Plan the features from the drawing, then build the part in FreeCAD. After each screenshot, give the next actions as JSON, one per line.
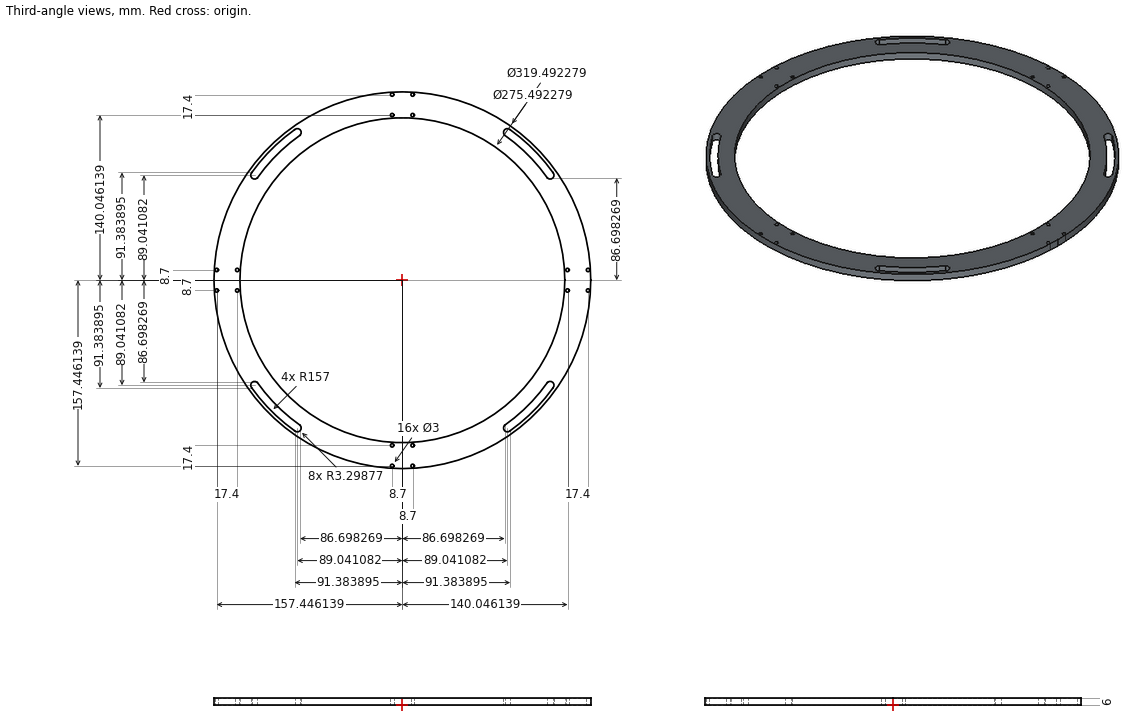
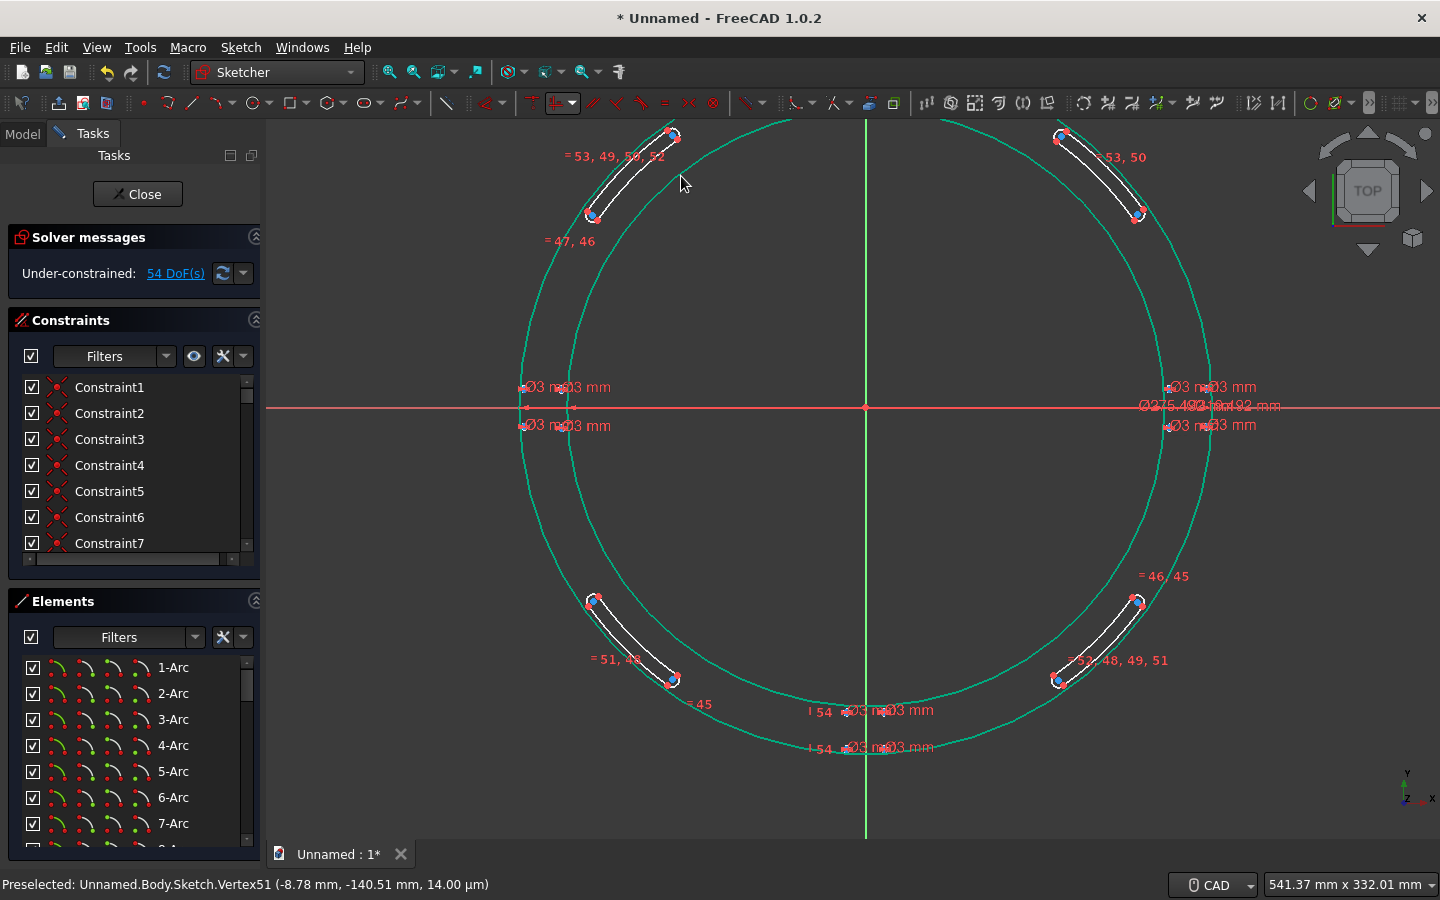
{"action": "left_click", "coordinate": [524, 427]}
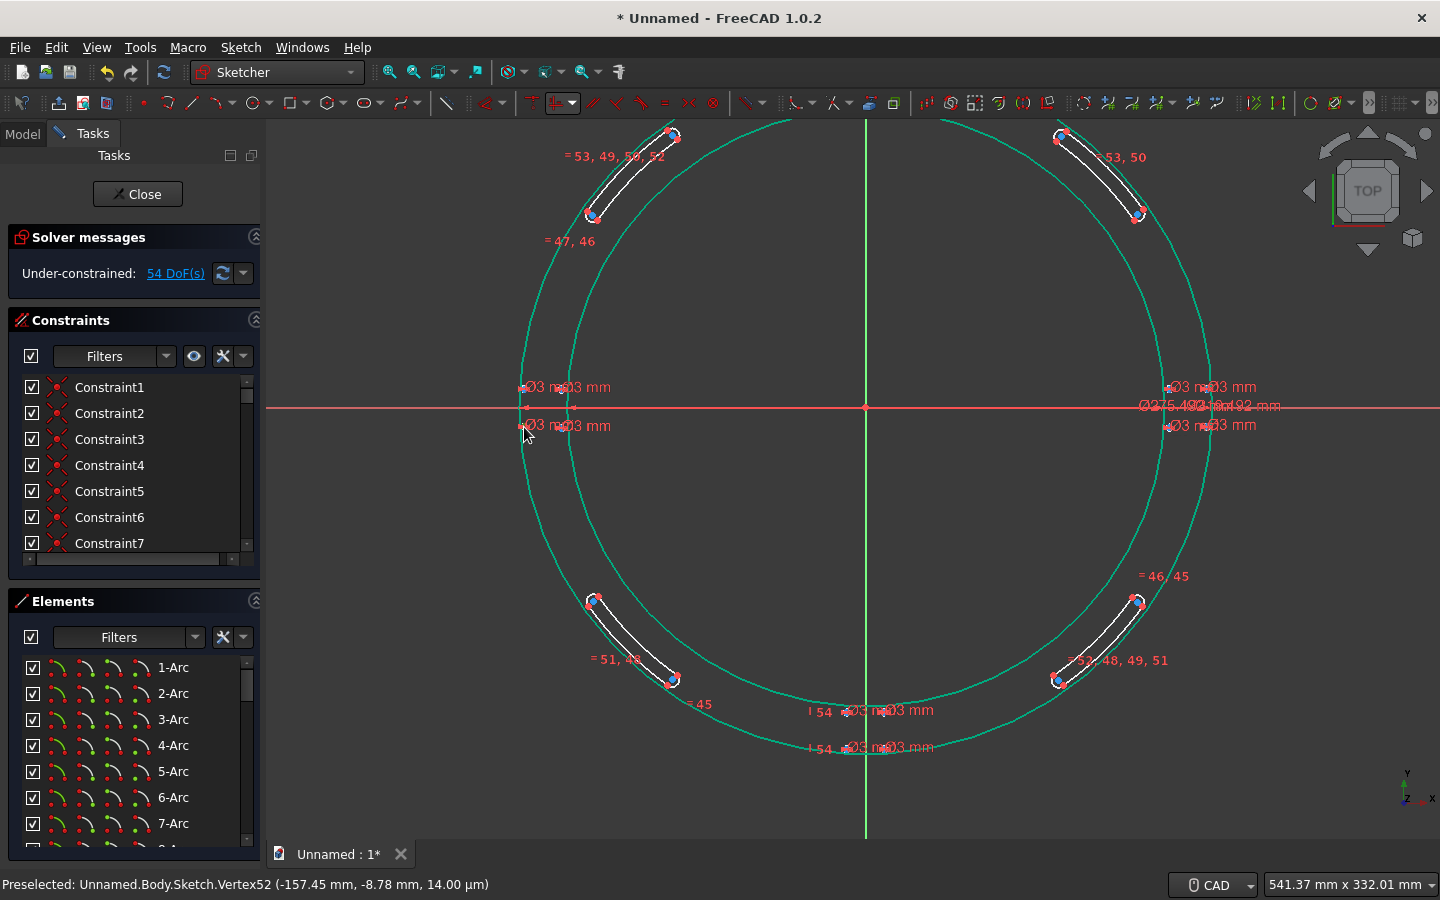
{"action": "left_click", "coordinate": [562, 428]}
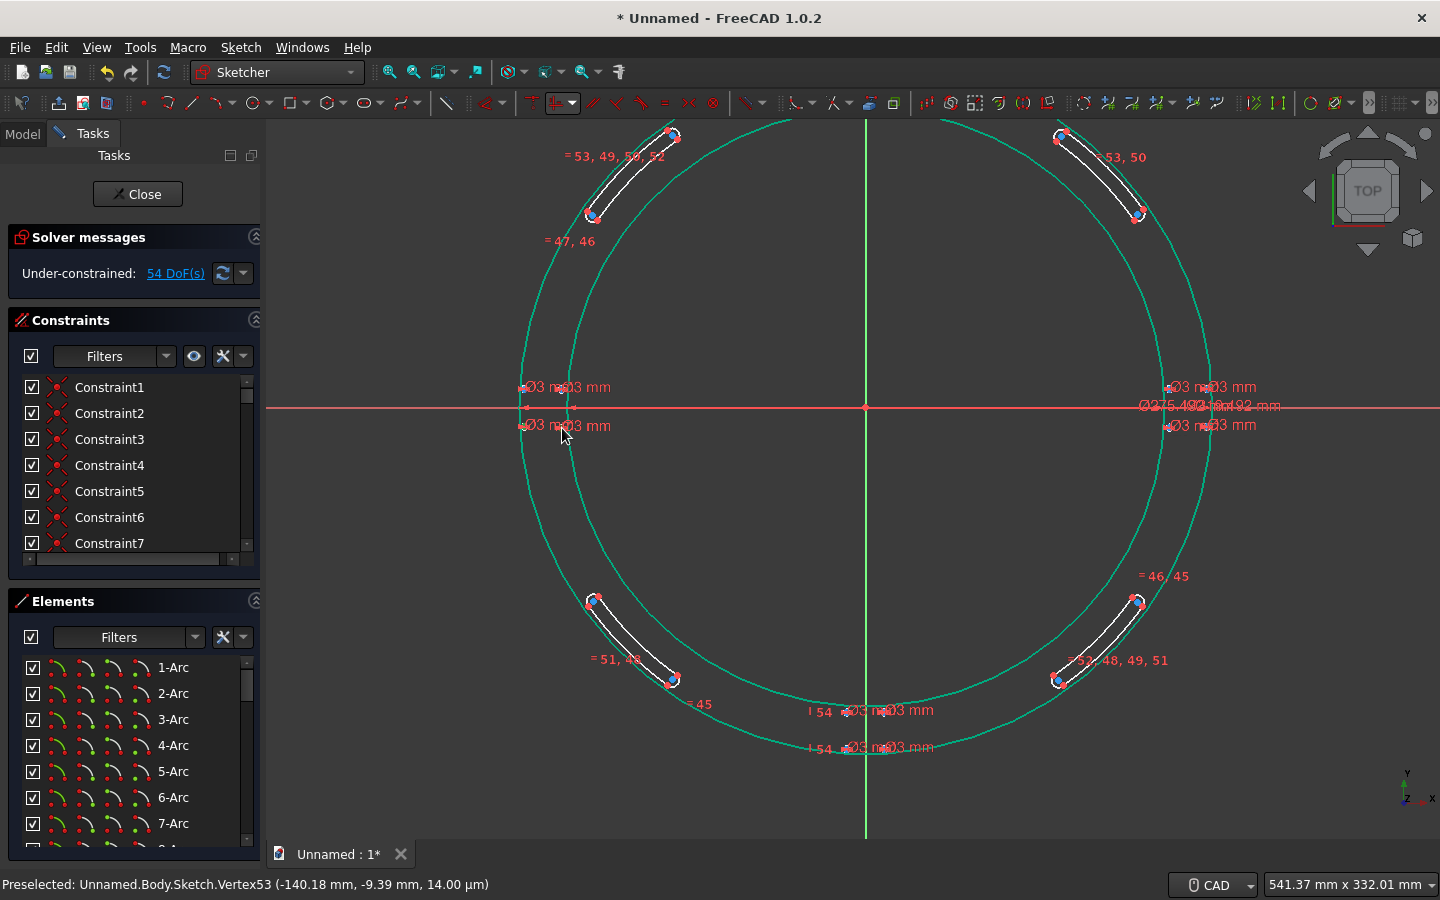
{"action": "key", "text": "h"}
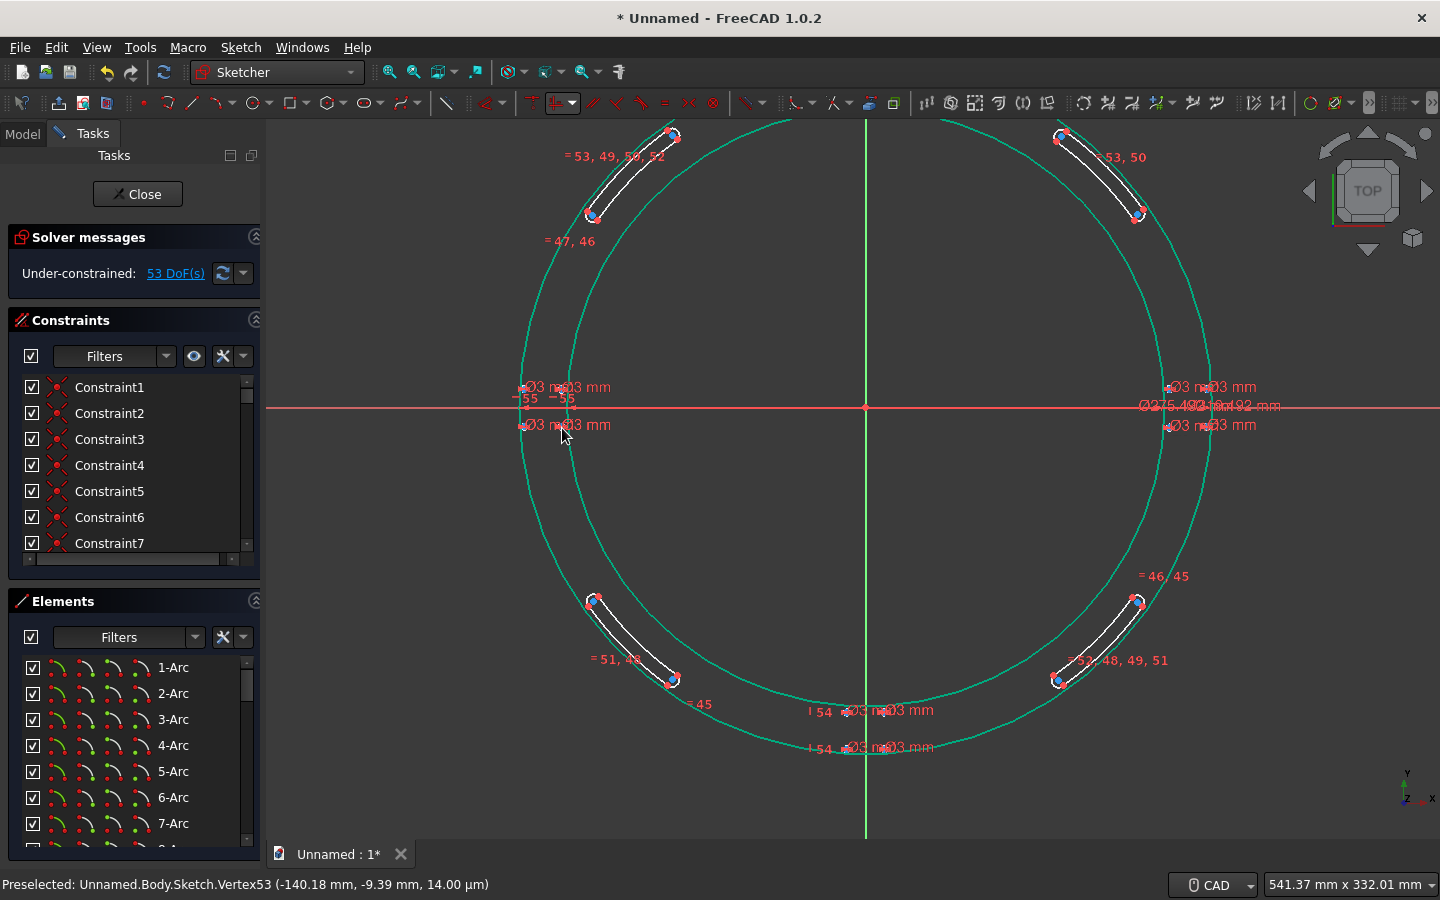
{"action": "left_click", "coordinate": [847, 749]}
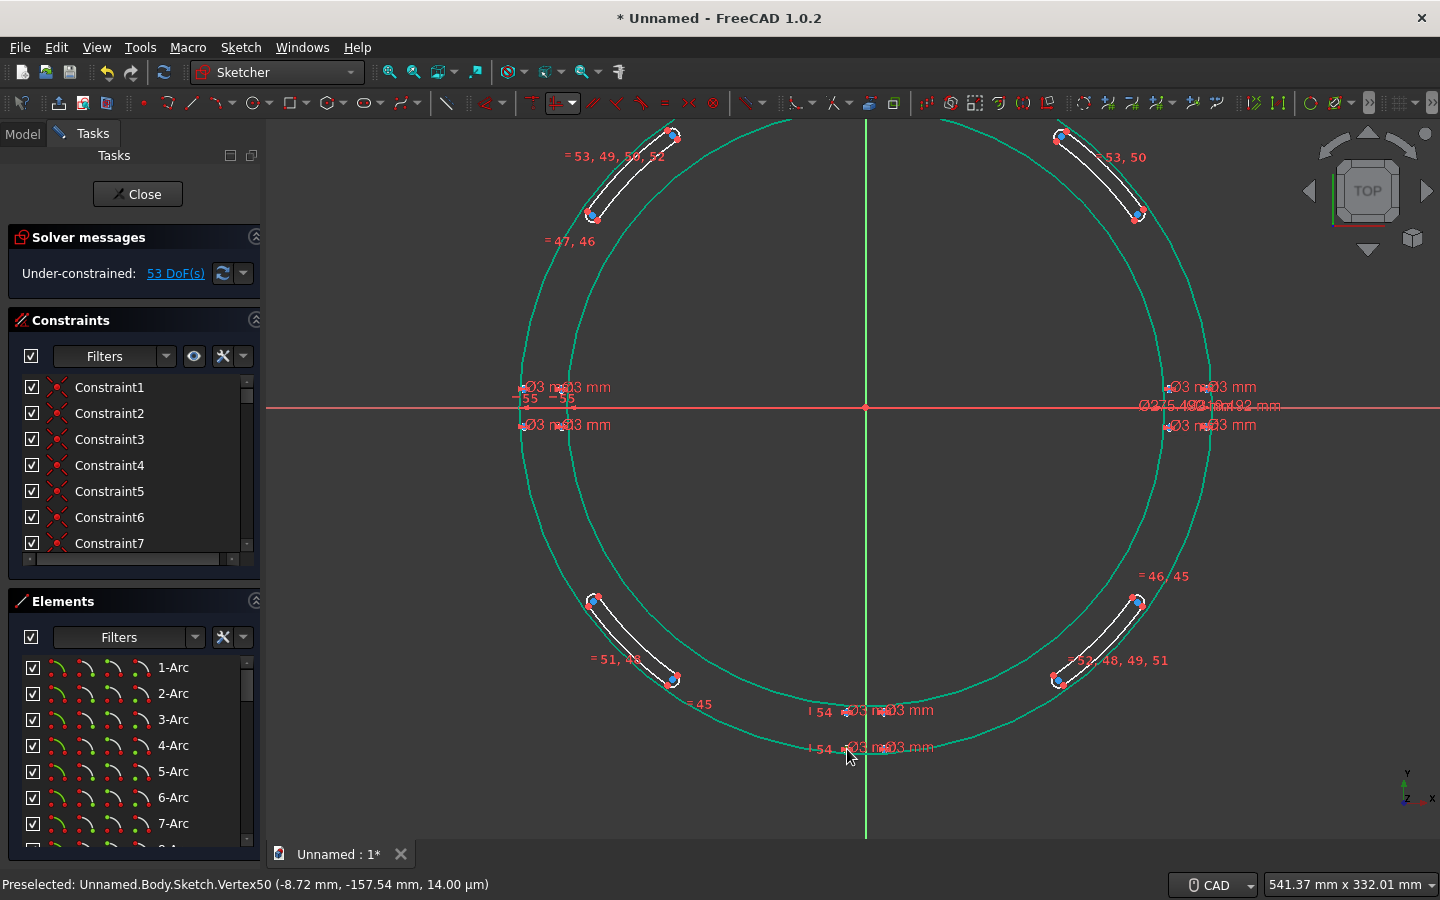
{"action": "left_click", "coordinate": [885, 749]}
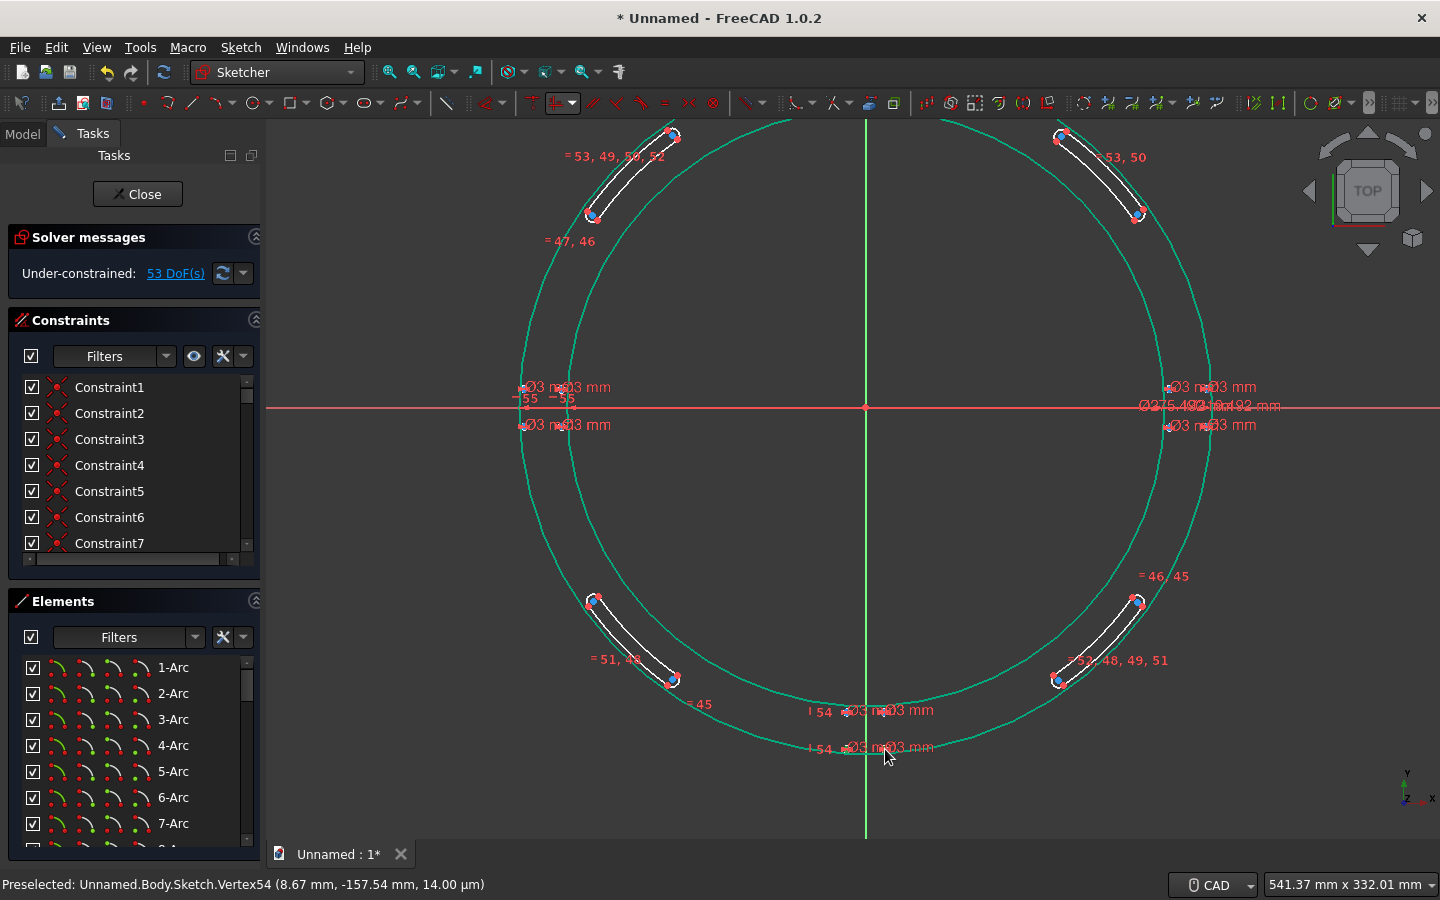
{"action": "key", "text": "h"}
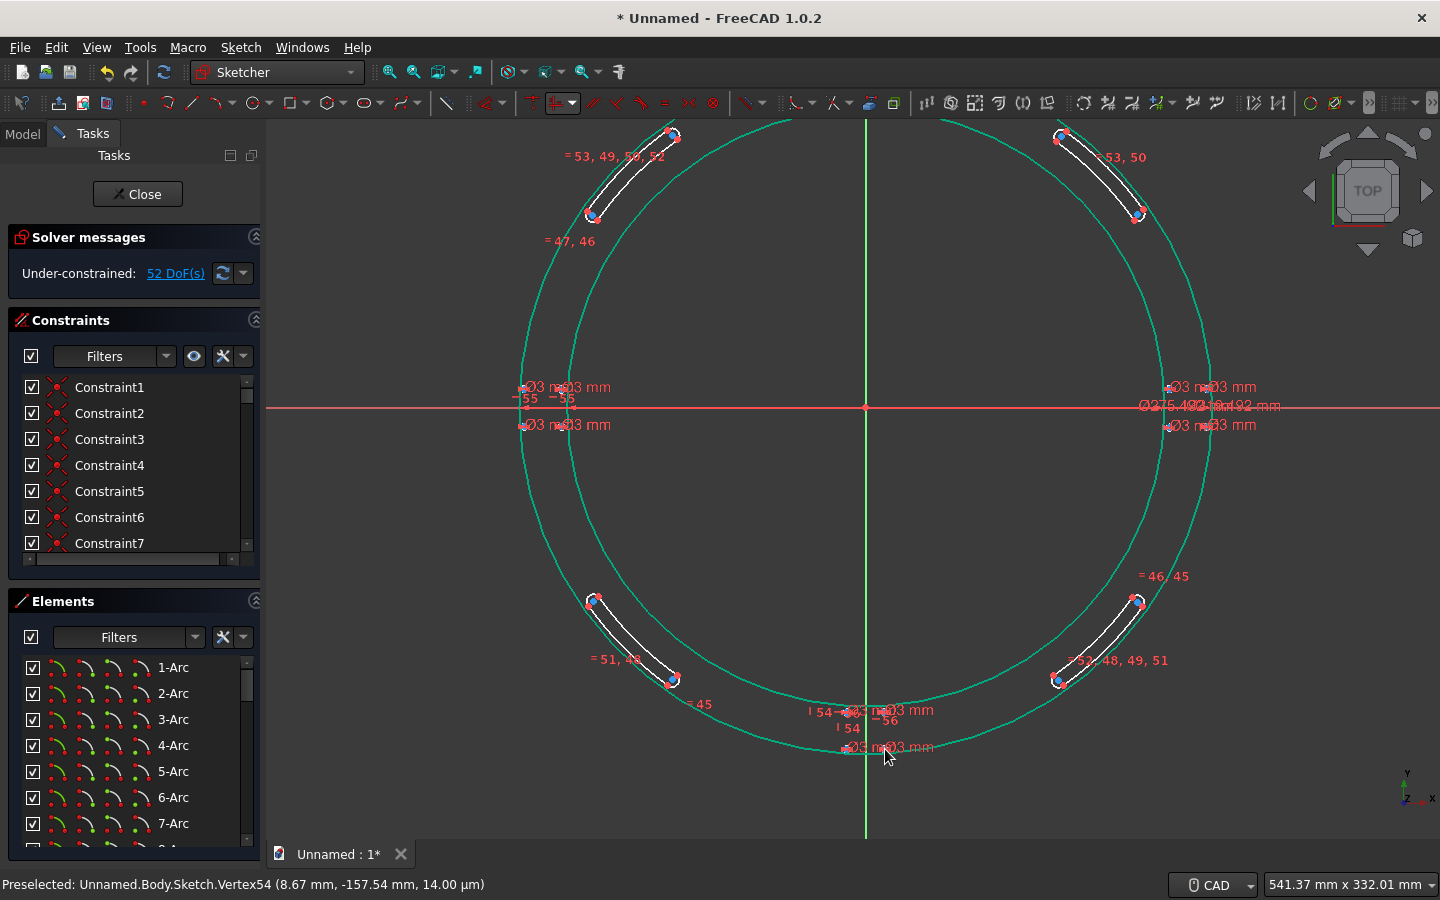
{"action": "left_click", "coordinate": [885, 749]}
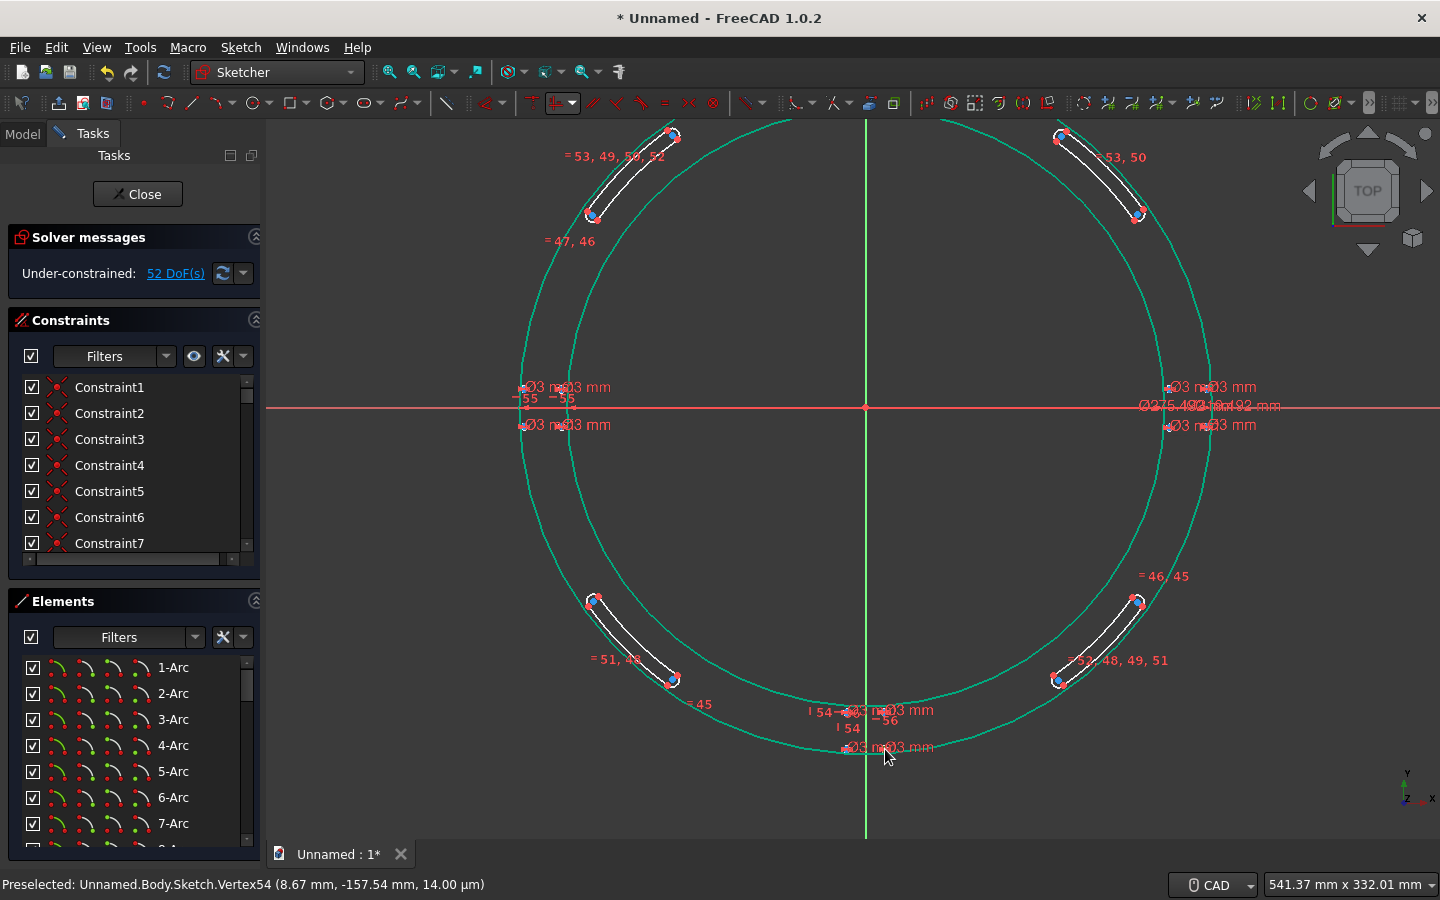
{"action": "left_click", "coordinate": [884, 712]}